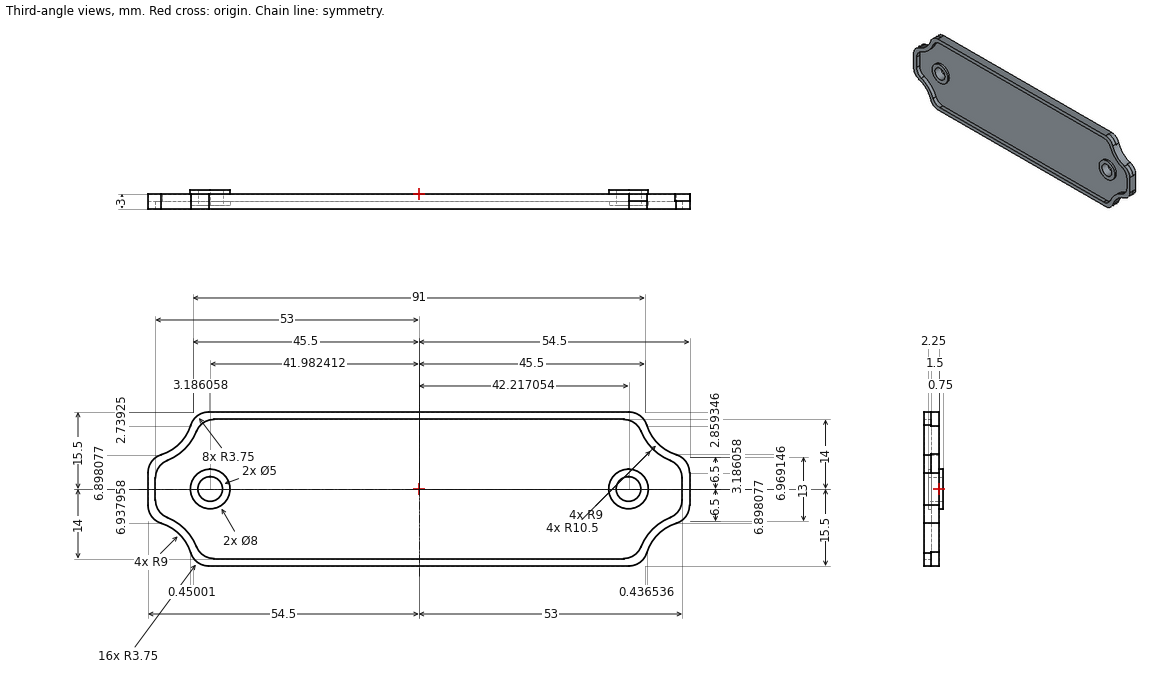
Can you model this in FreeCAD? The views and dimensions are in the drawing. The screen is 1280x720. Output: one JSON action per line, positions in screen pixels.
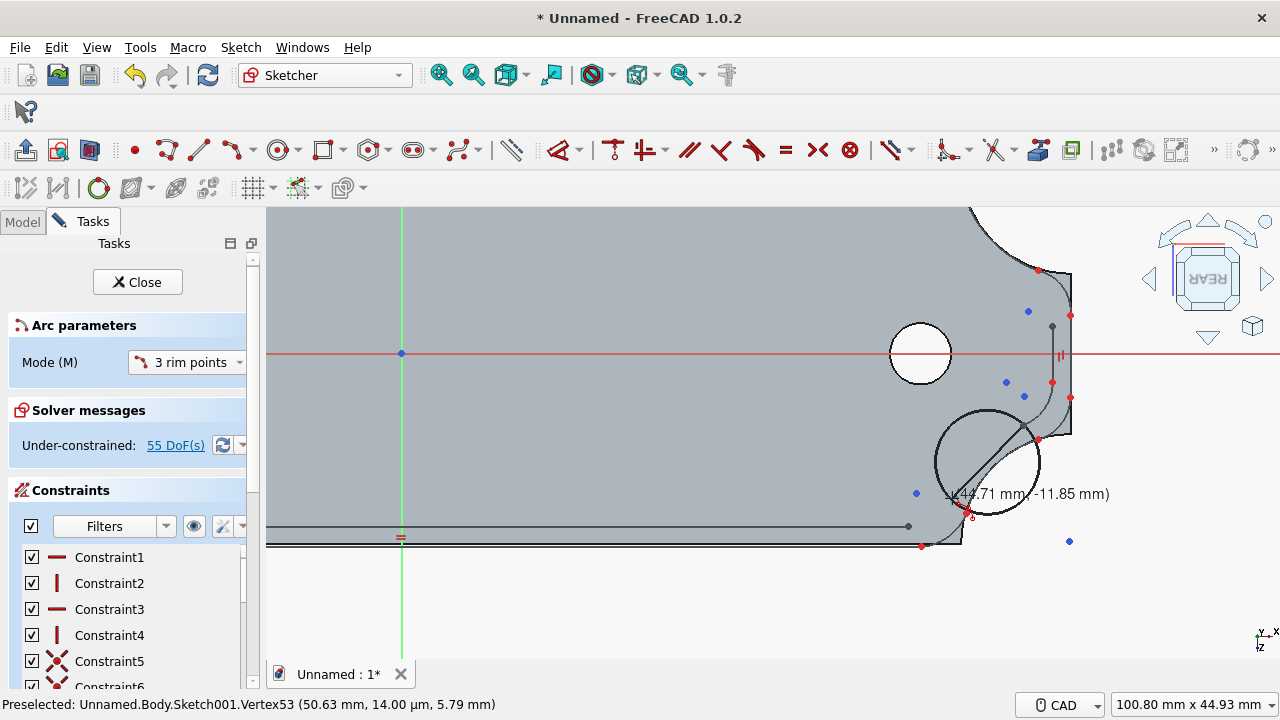
{"action": "left_click", "coordinate": [952, 497]}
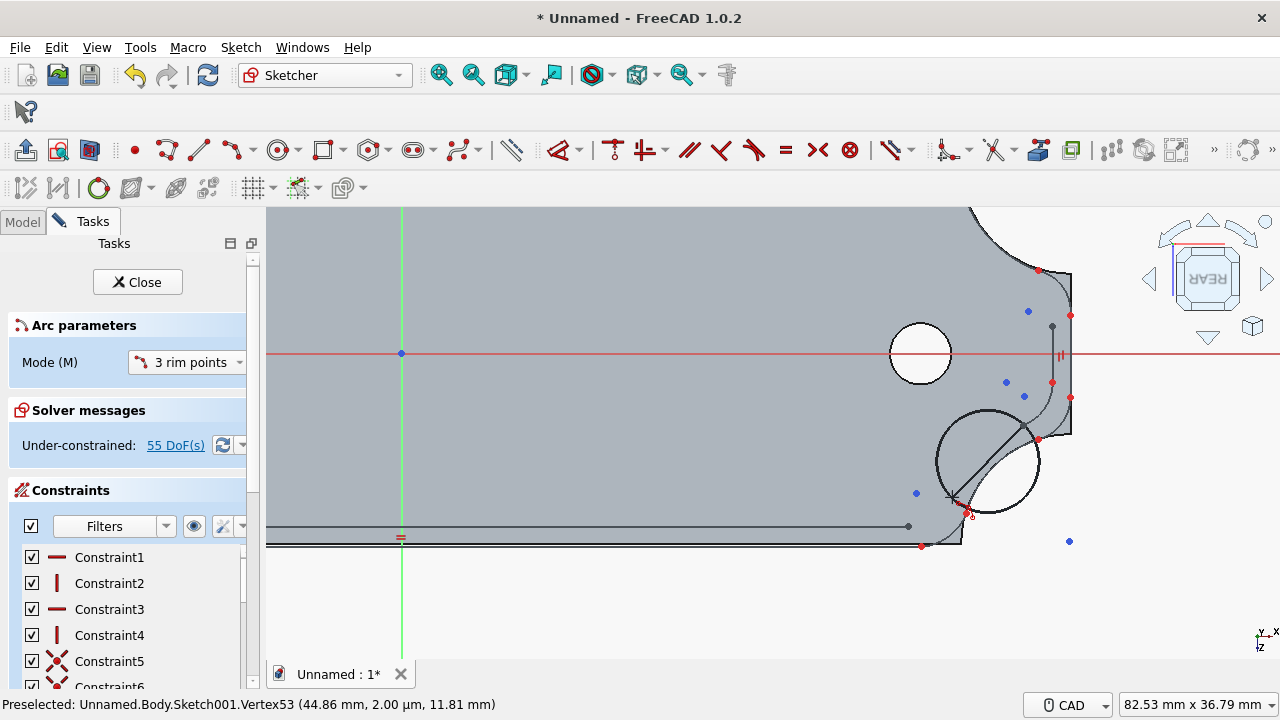
{"action": "scroll", "coordinate": [980, 453], "scroll_direction": "up", "scroll_amount": 3}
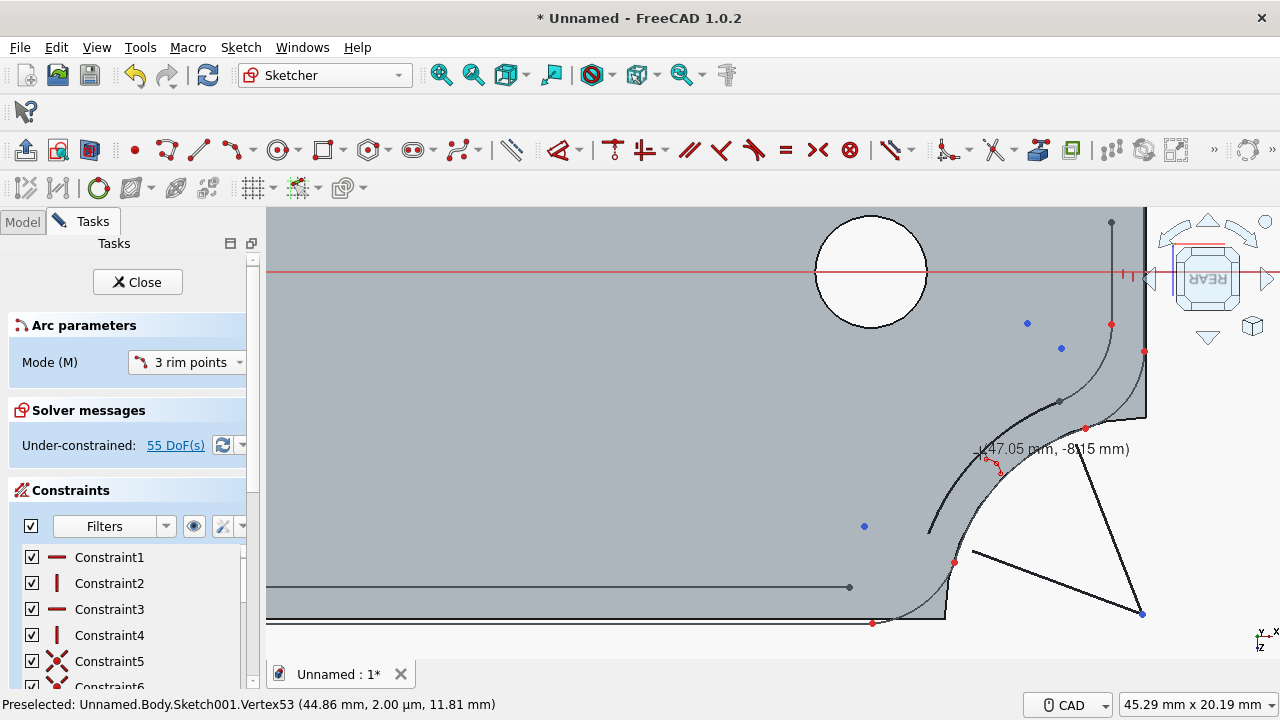
{"action": "left_click", "coordinate": [980, 453]}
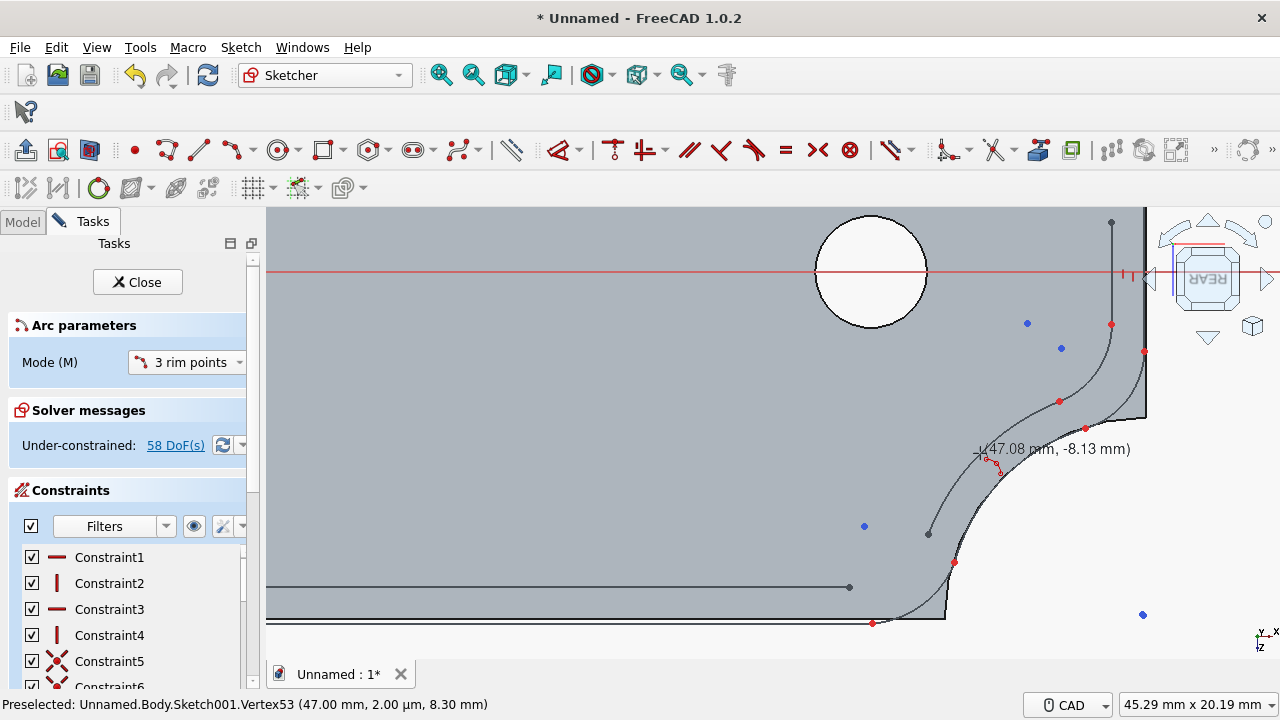
{"action": "left_click", "coordinate": [928, 535]}
{"action": "left_click", "coordinate": [849, 587]}
{"action": "left_click", "coordinate": [897, 571]}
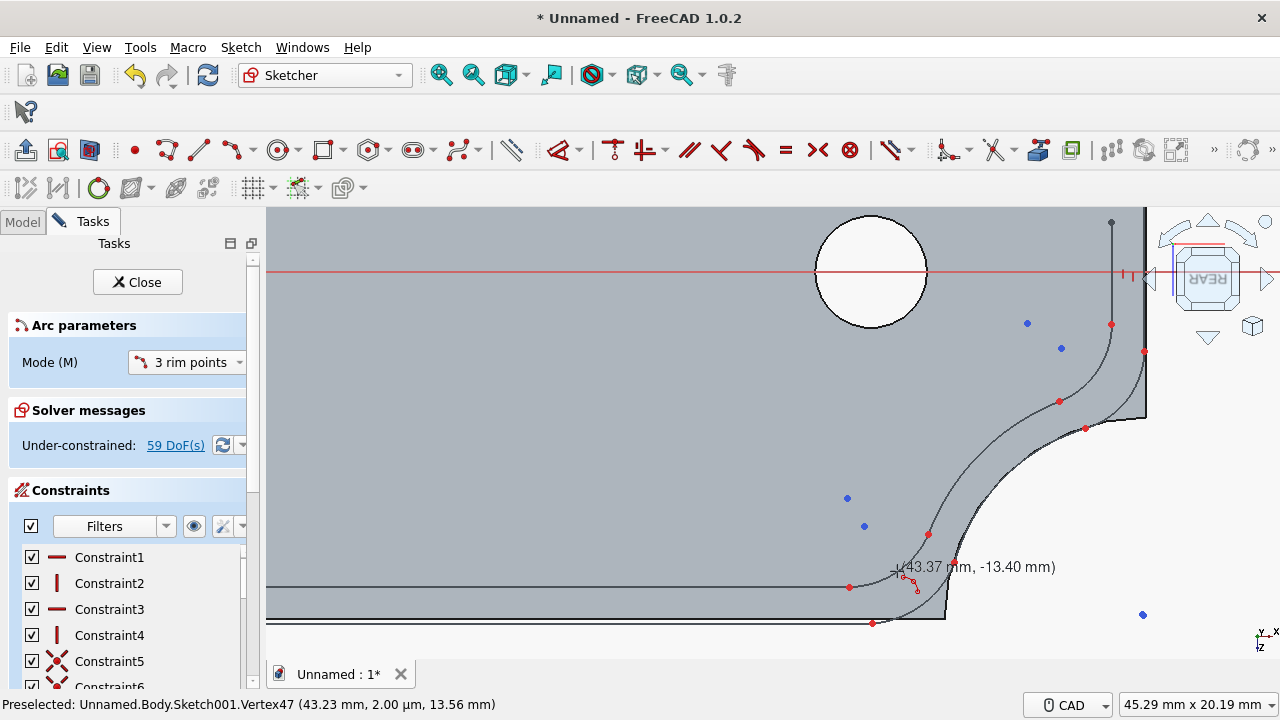
{"action": "scroll", "coordinate": [959, 486], "scroll_direction": "down", "scroll_amount": 7}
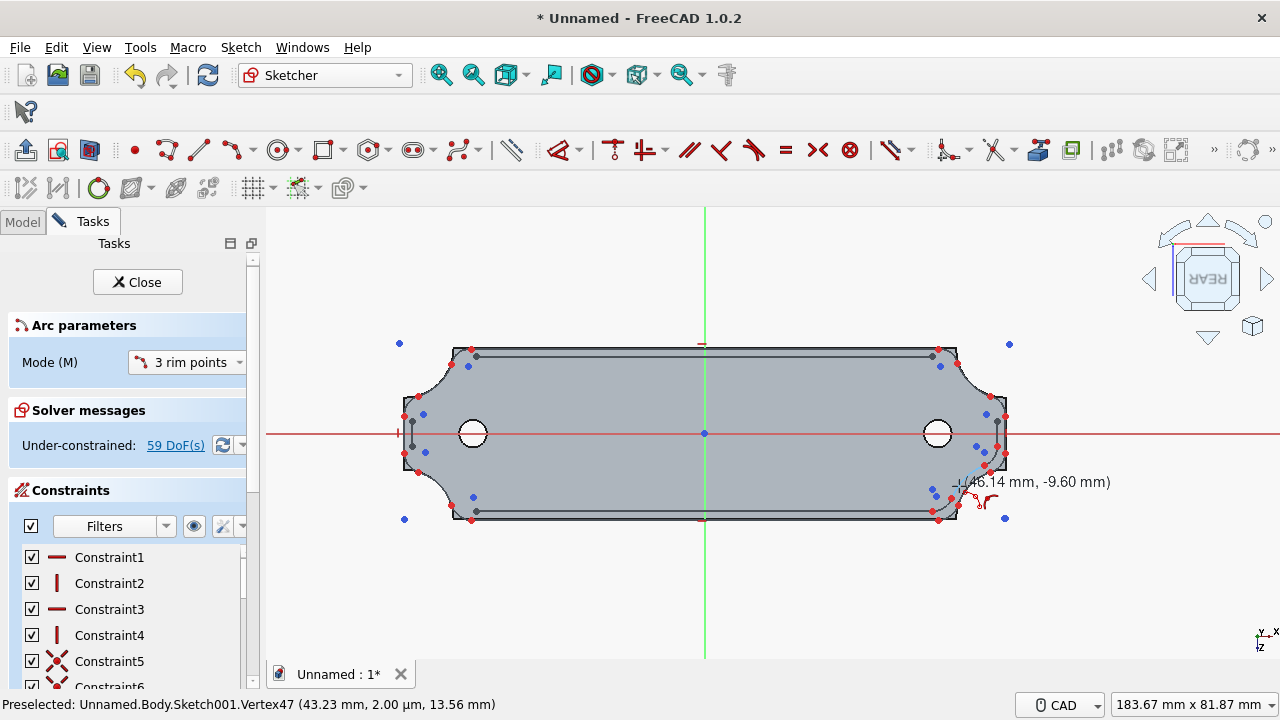
{"action": "scroll", "coordinate": [477, 511], "scroll_direction": "up", "scroll_amount": 4}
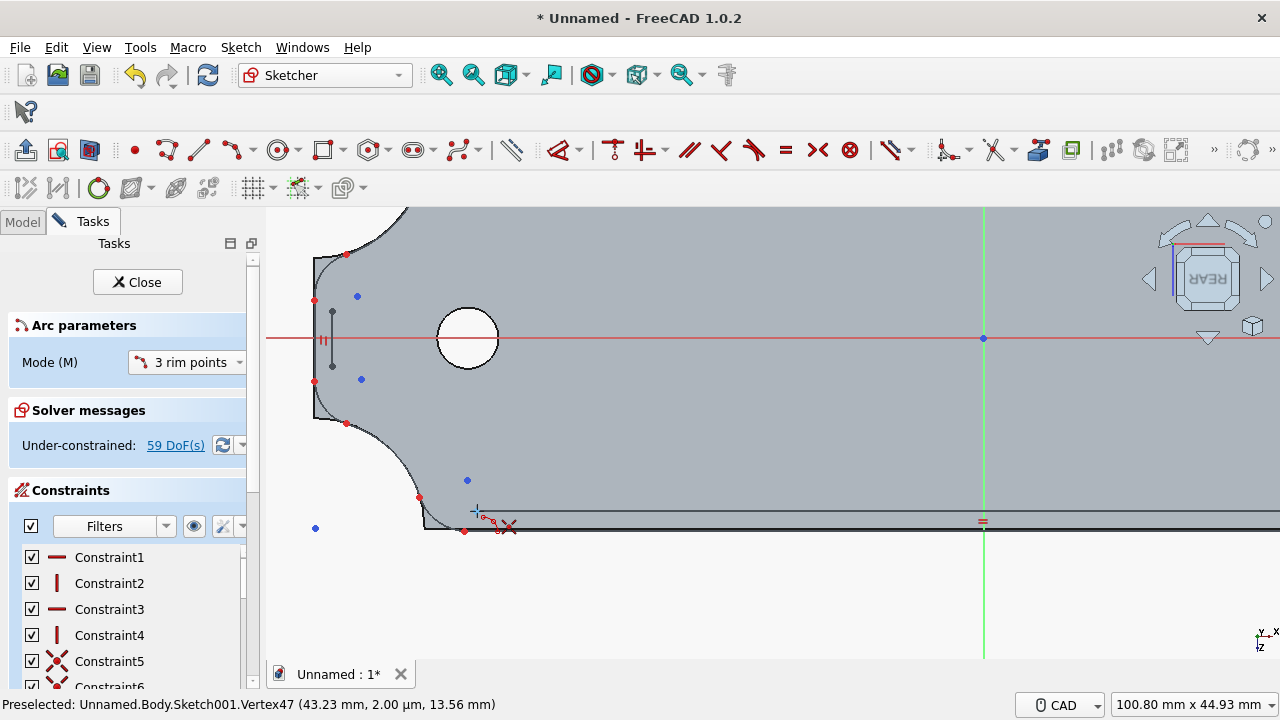
{"action": "left_click", "coordinate": [476, 511]}
{"action": "left_click", "coordinate": [434, 481]}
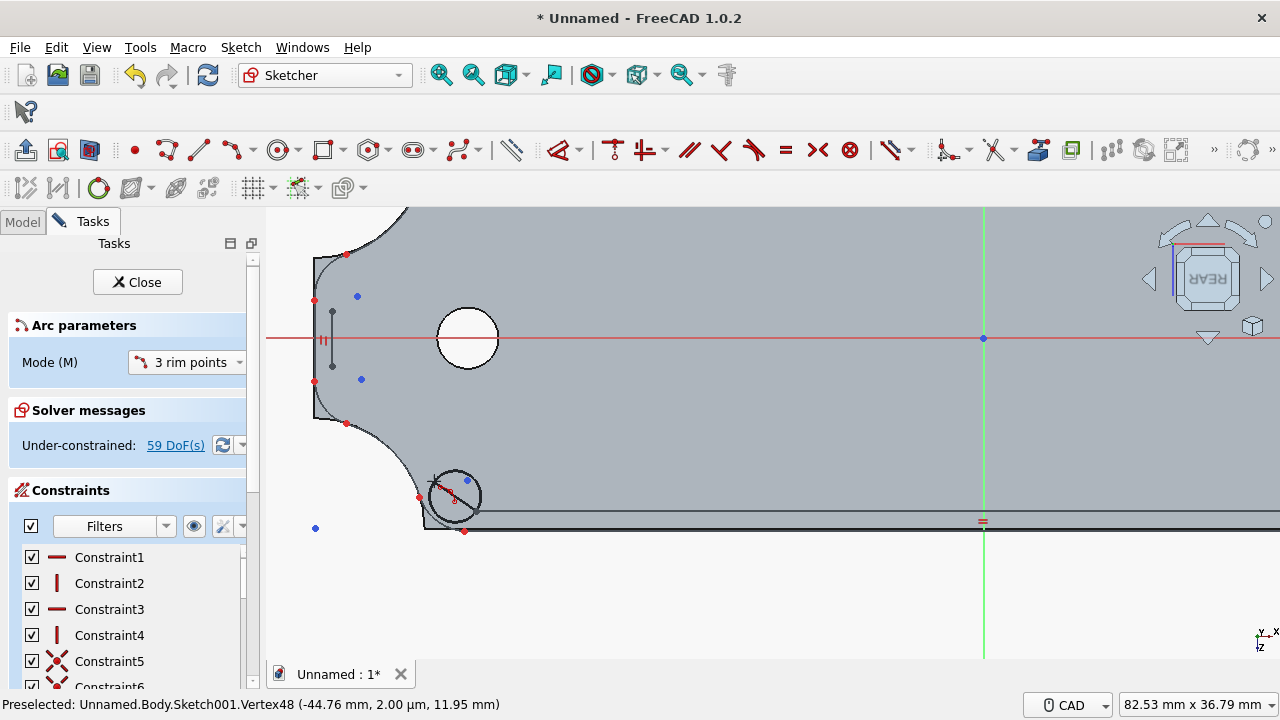
{"action": "scroll", "coordinate": [451, 502], "scroll_direction": "up", "scroll_amount": 4}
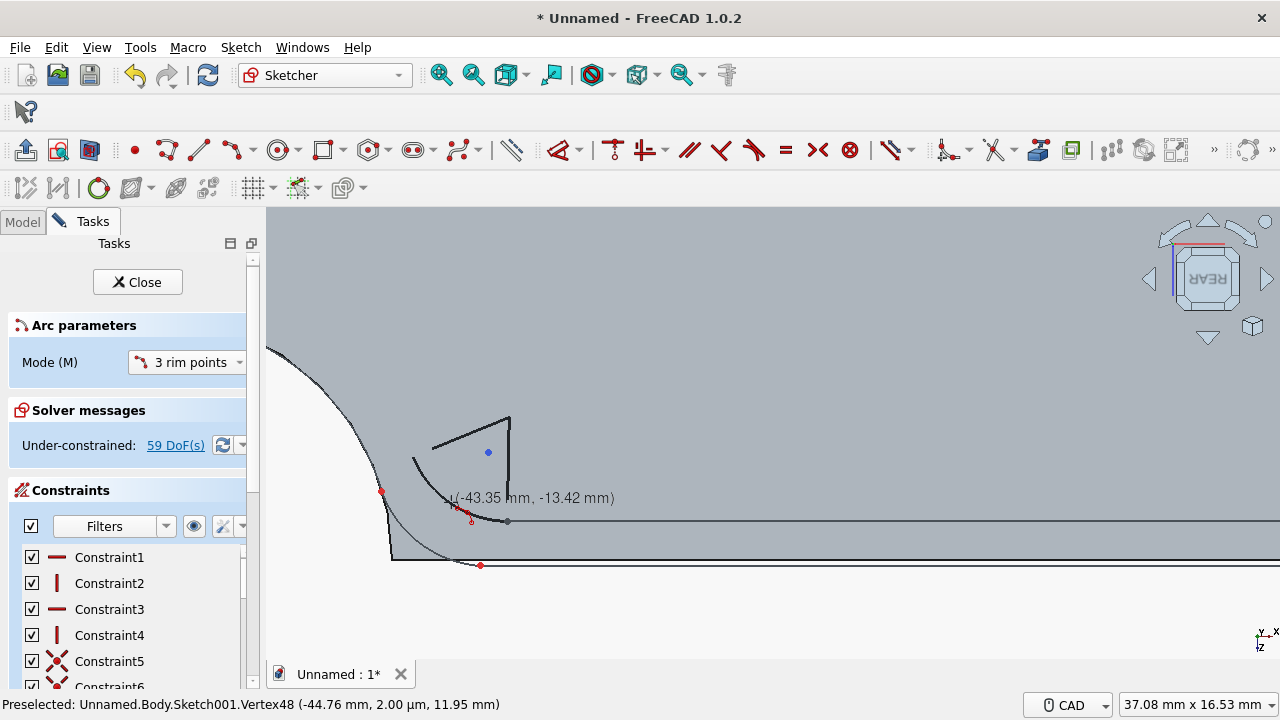
{"action": "left_click", "coordinate": [451, 502]}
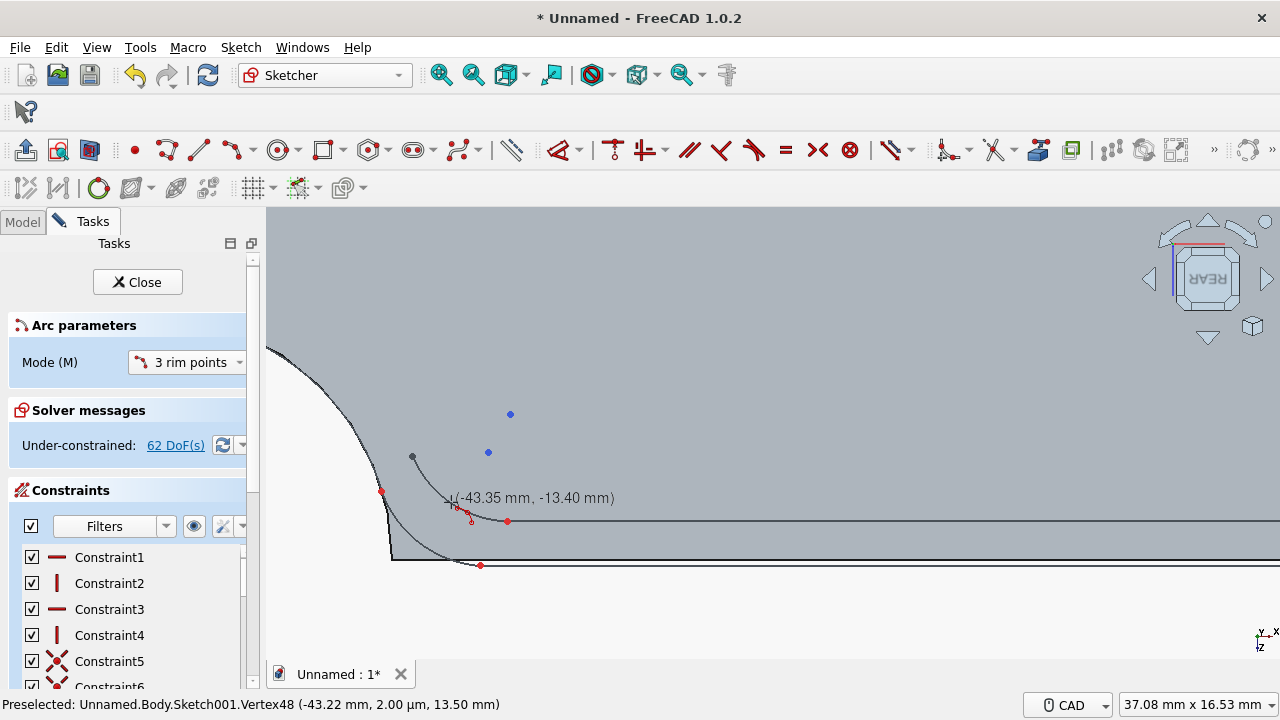
{"action": "left_click", "coordinate": [413, 457]}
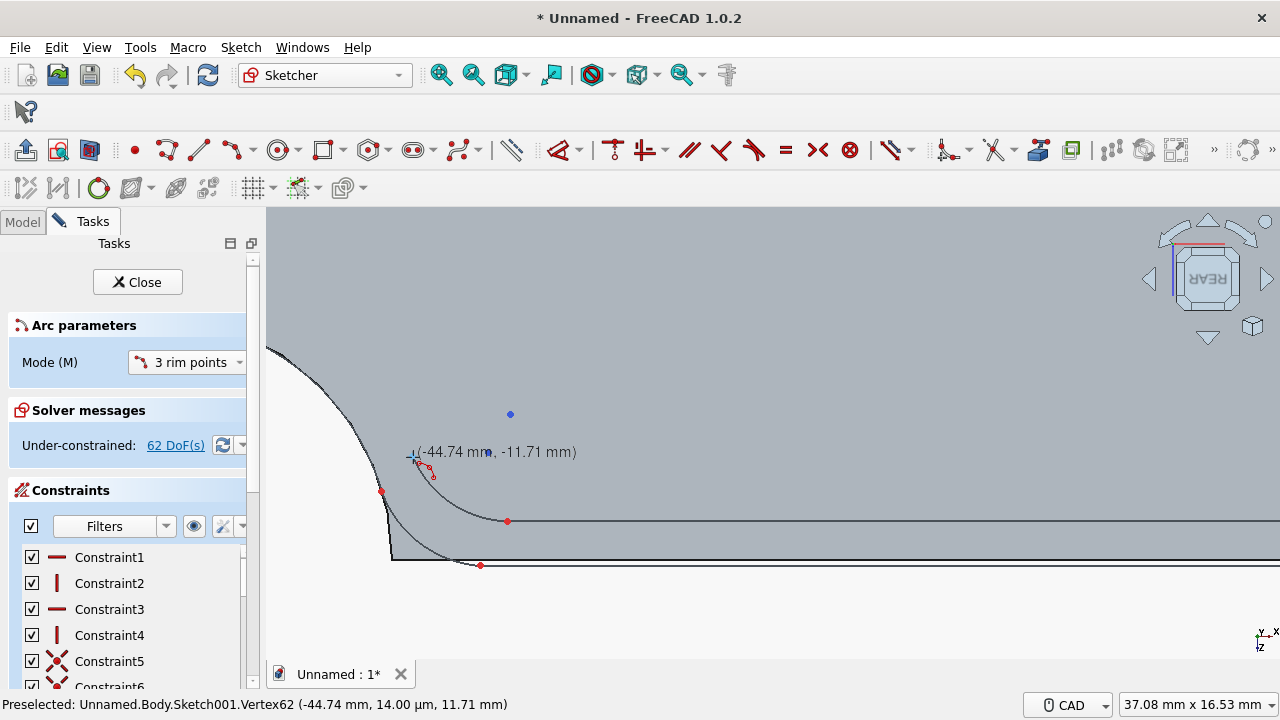
{"action": "scroll", "coordinate": [469, 508], "scroll_direction": "down", "scroll_amount": 8}